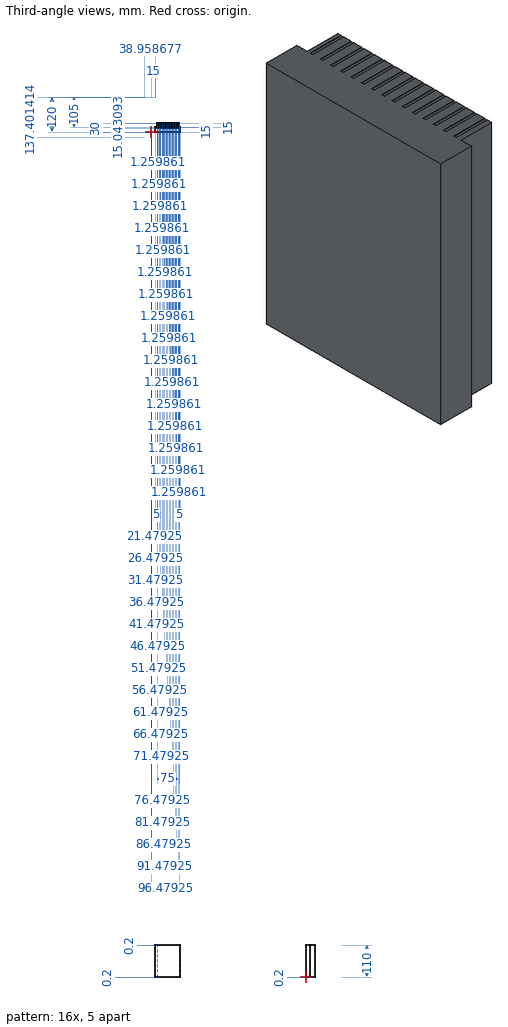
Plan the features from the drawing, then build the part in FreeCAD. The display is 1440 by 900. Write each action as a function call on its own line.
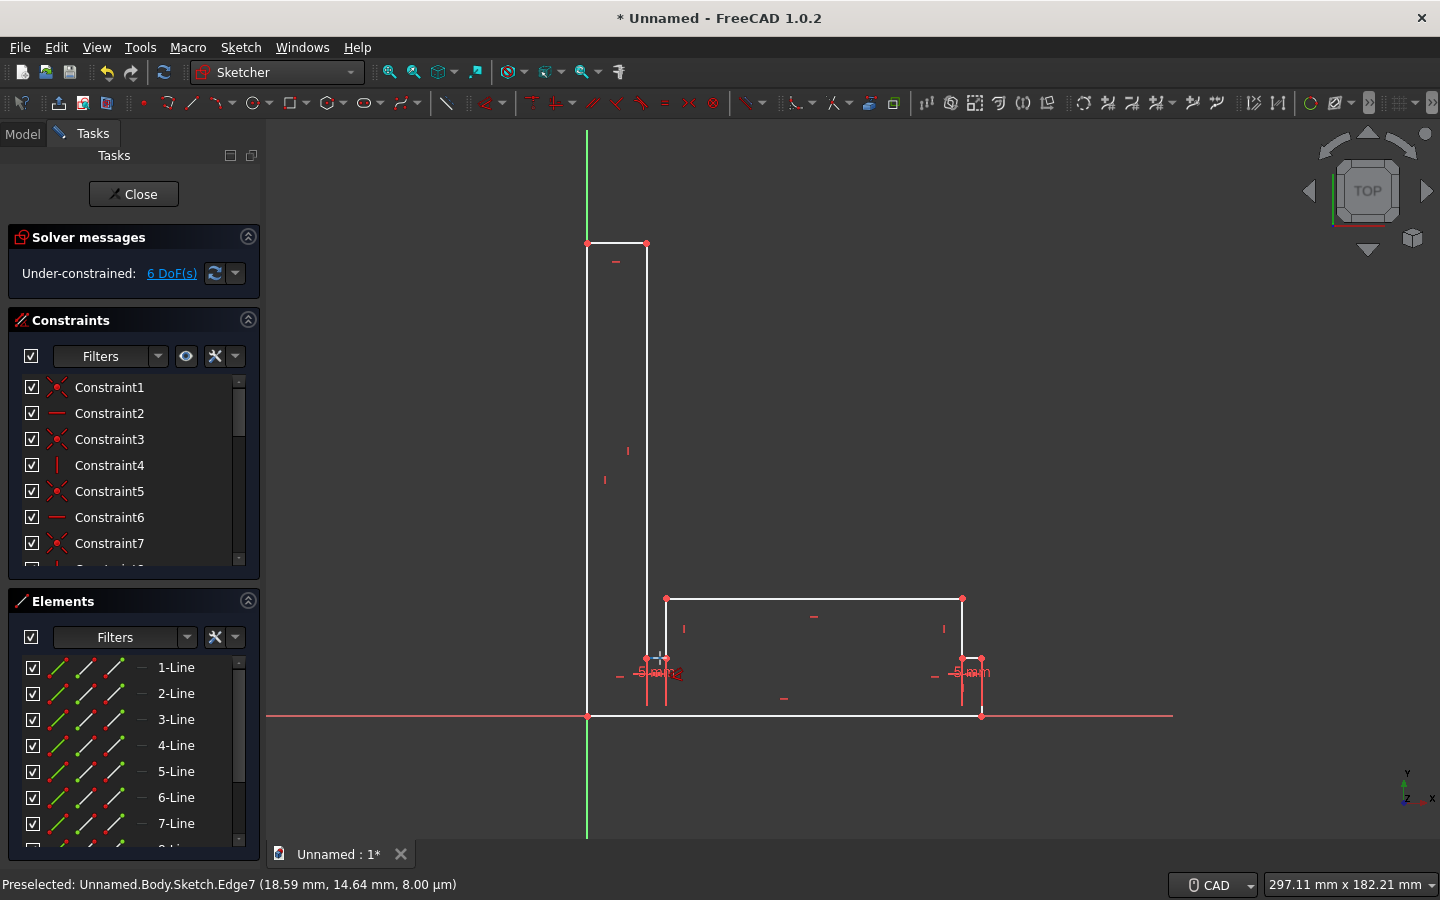
click(982, 699)
click(1016, 701)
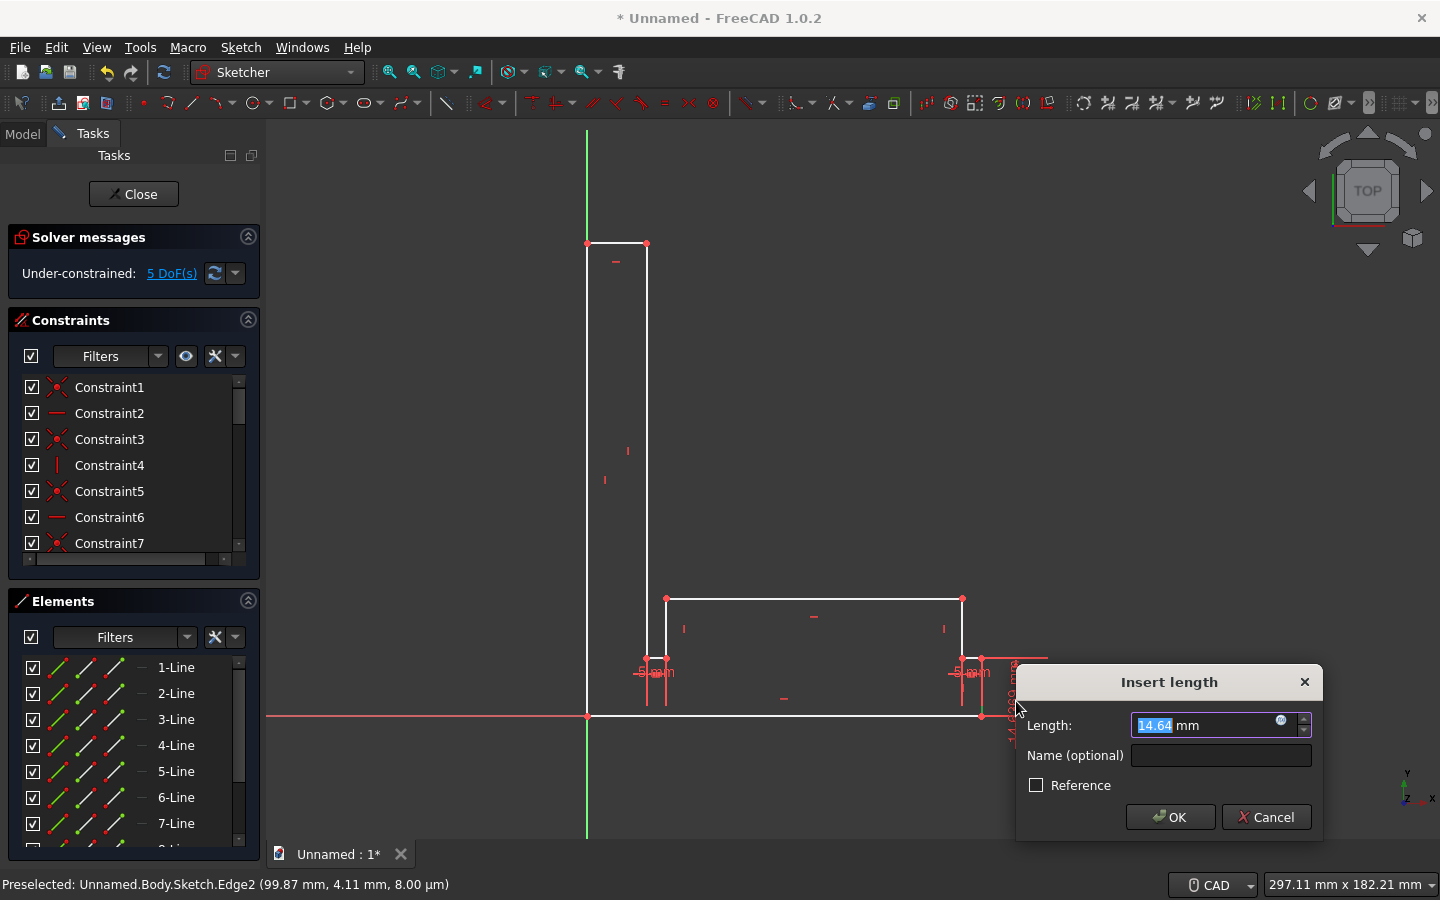
text(15)
key(Return)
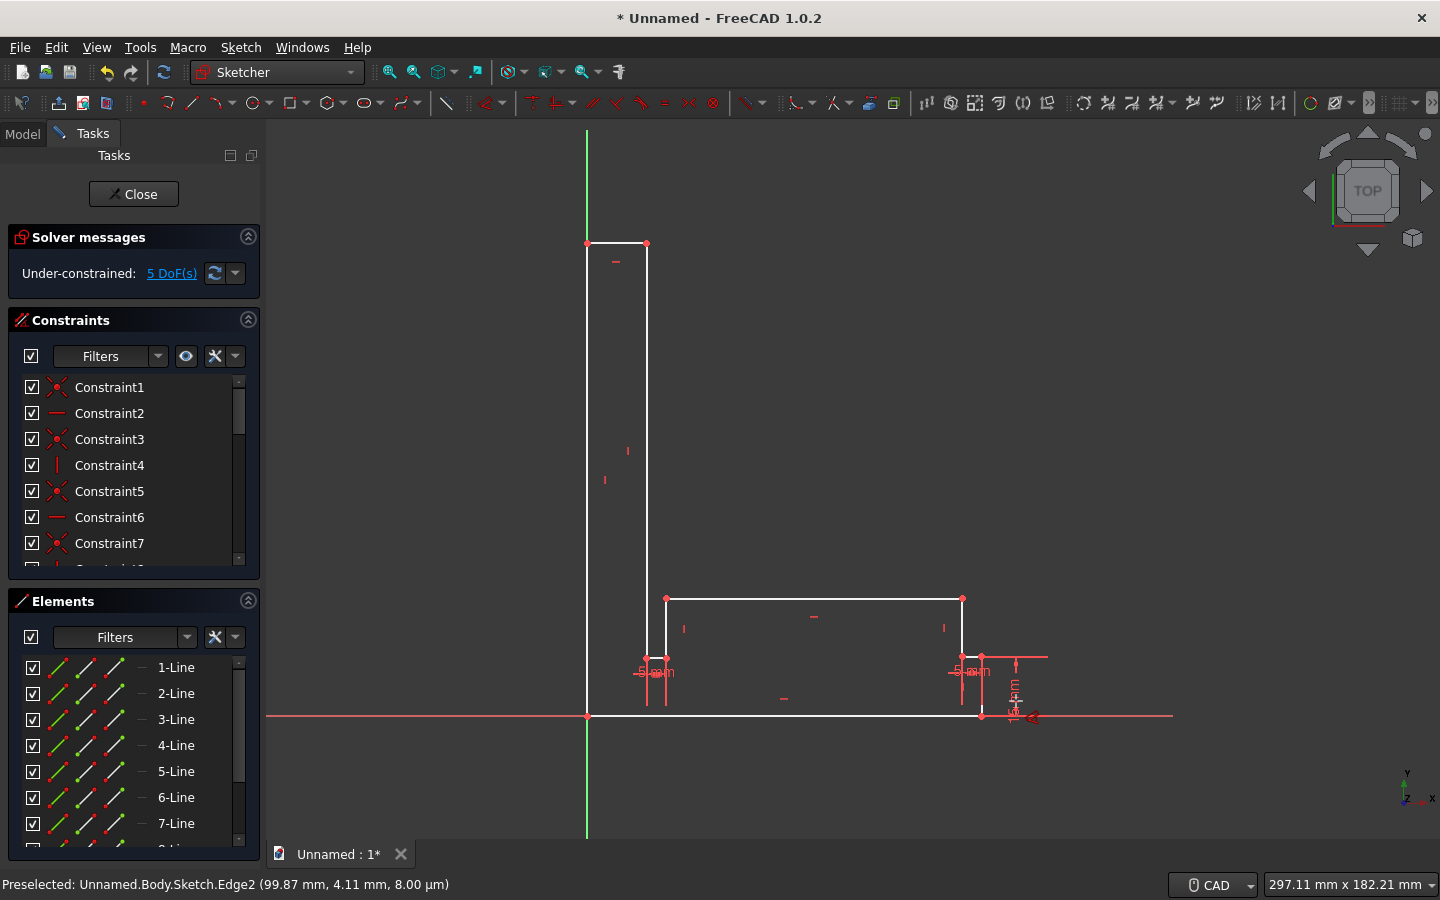
click(962, 639)
click(996, 628)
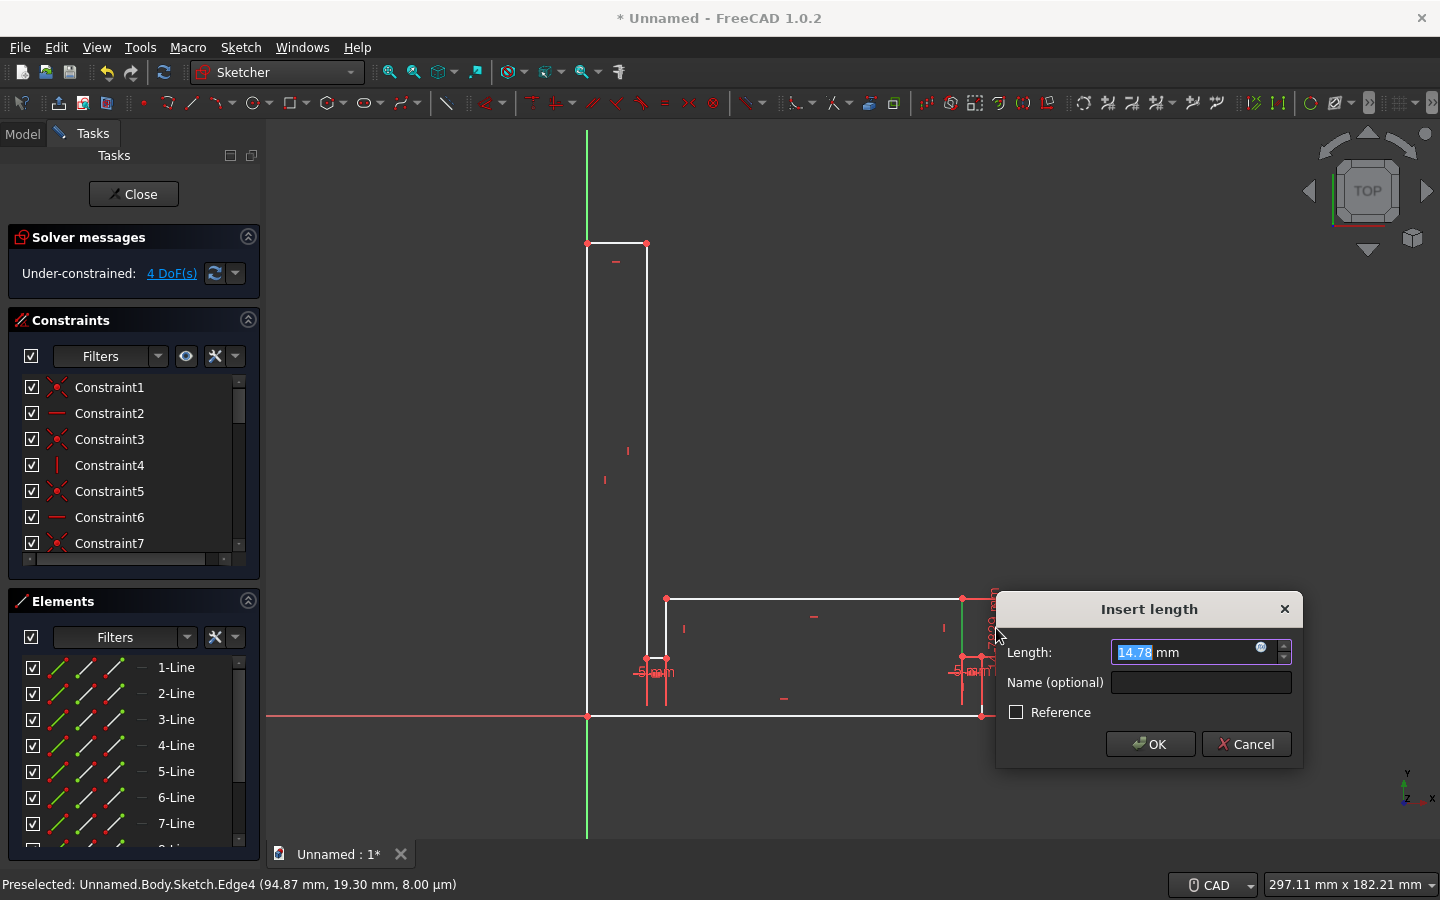
text(15)
key(Return)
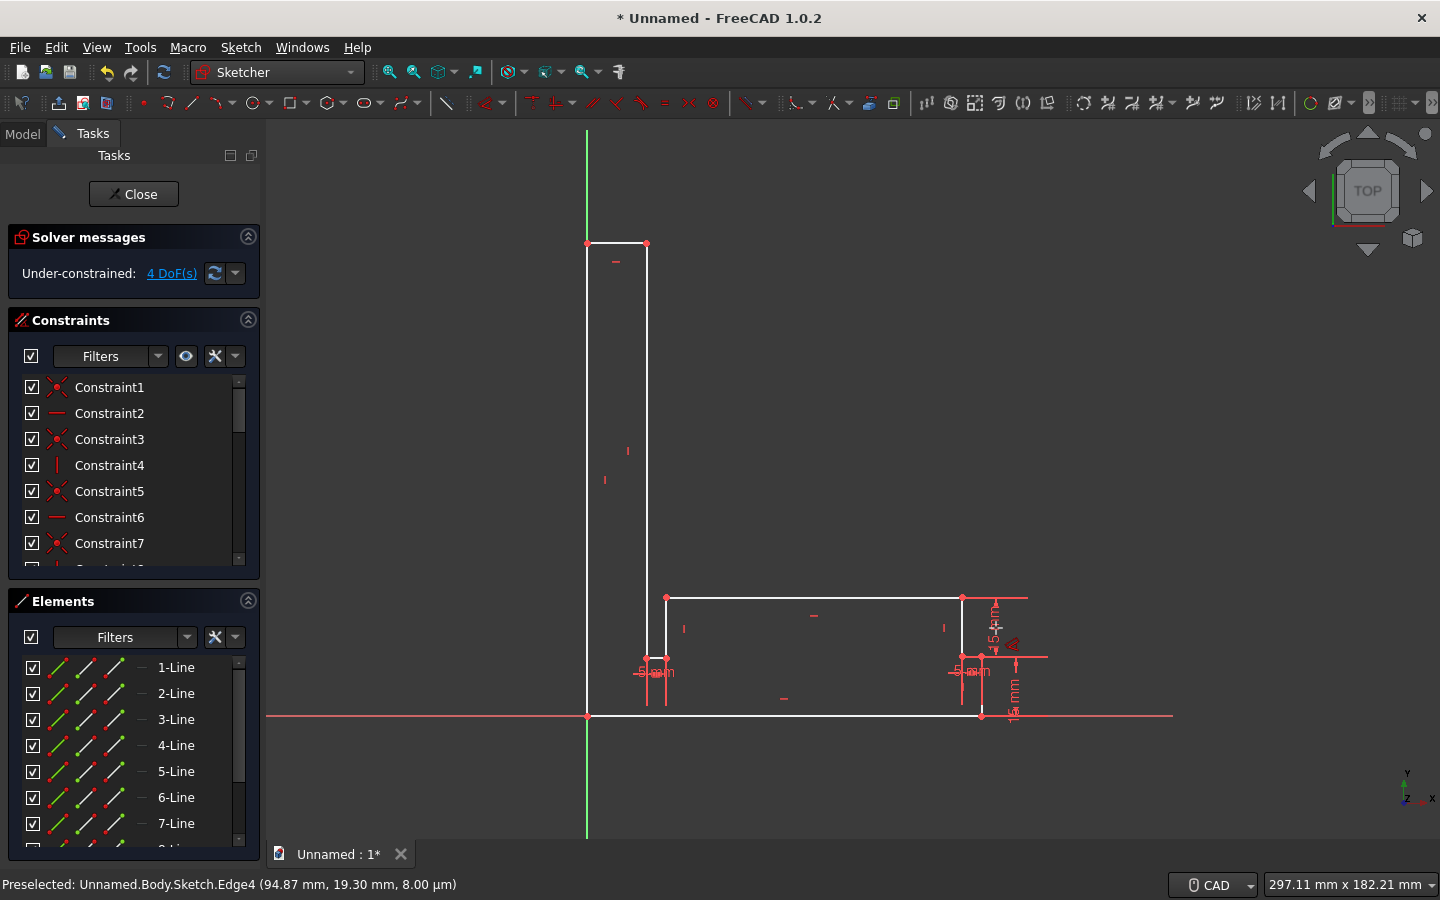
click(873, 598)
click(814, 632)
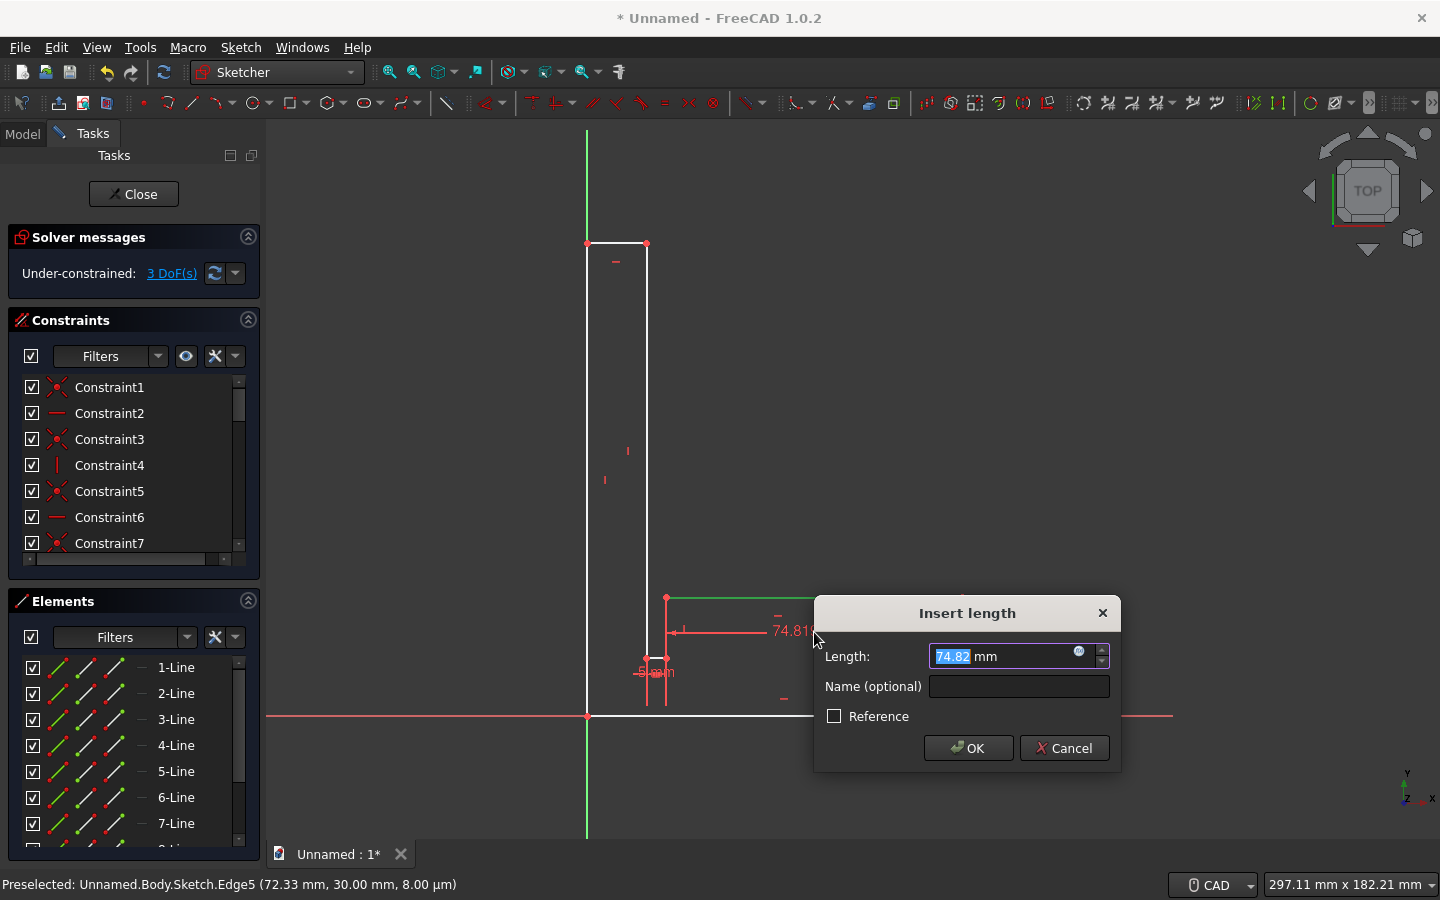
text(75)
key(Return)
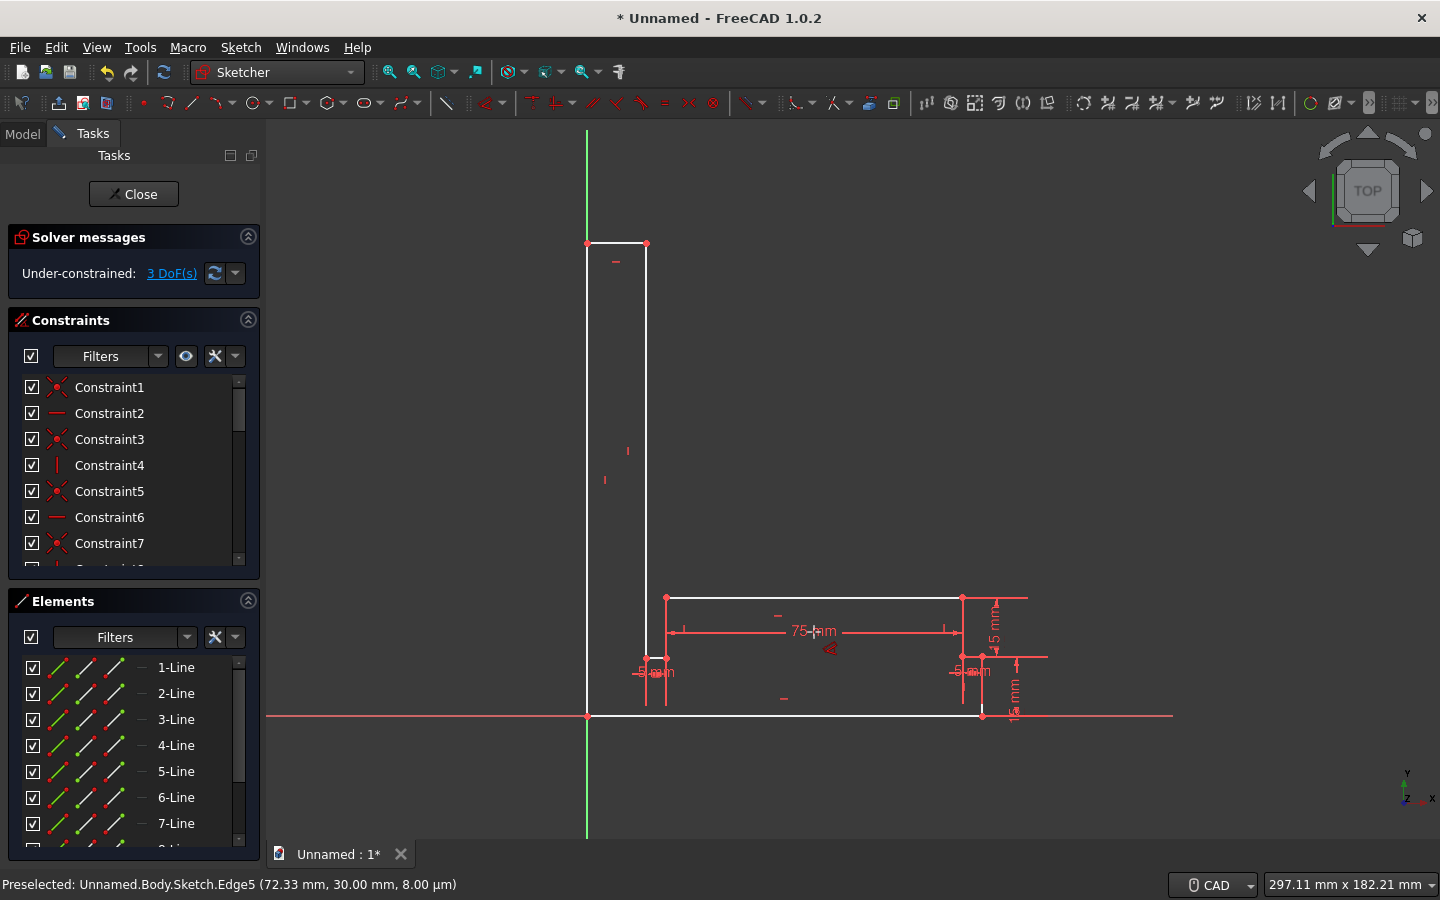
click(666, 616)
click(632, 628)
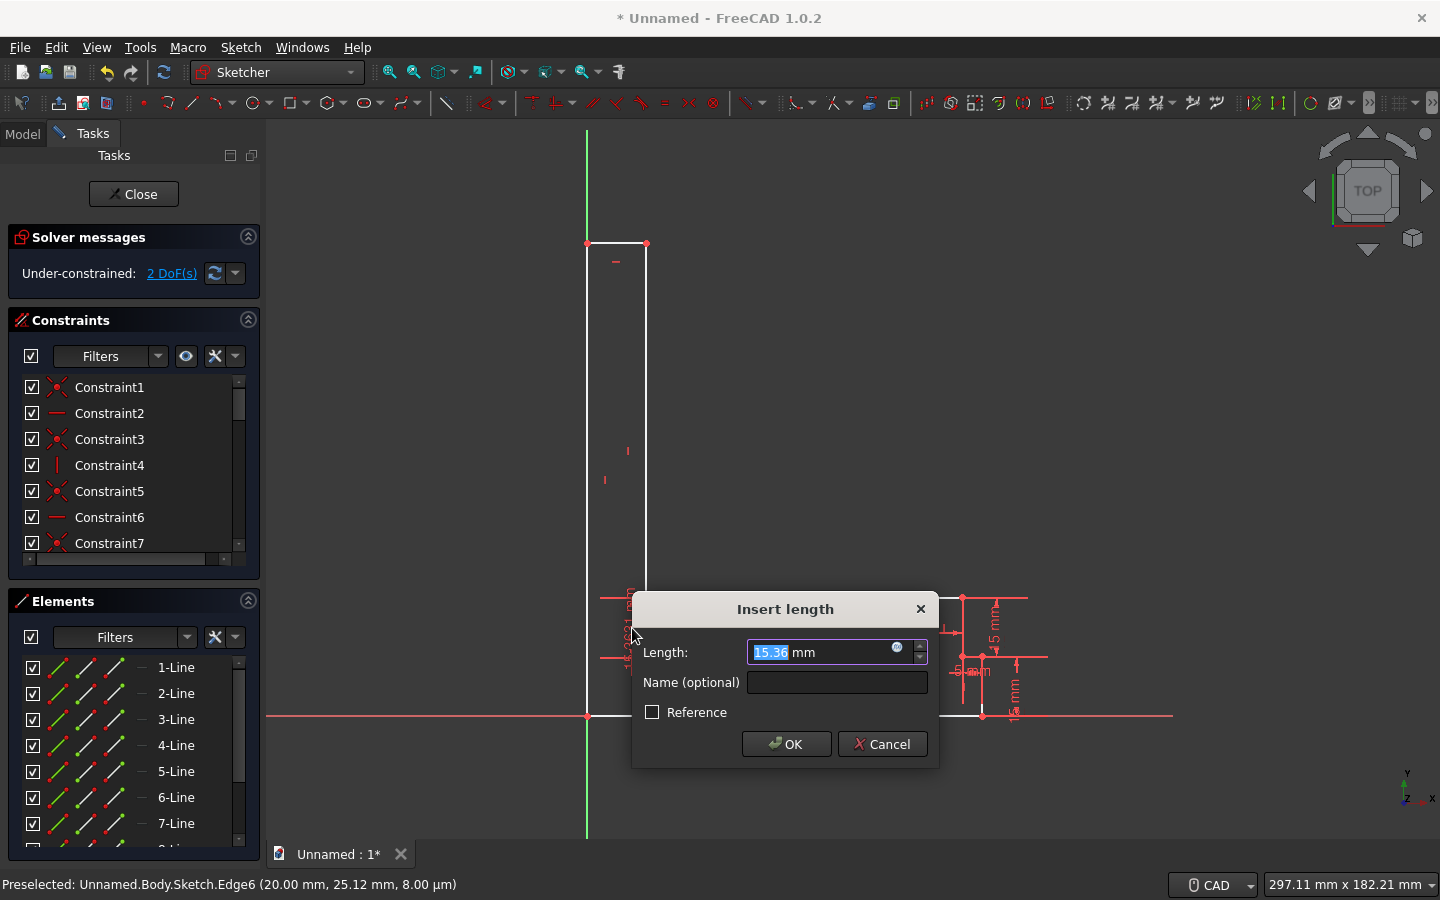
text(15)
key(Return)